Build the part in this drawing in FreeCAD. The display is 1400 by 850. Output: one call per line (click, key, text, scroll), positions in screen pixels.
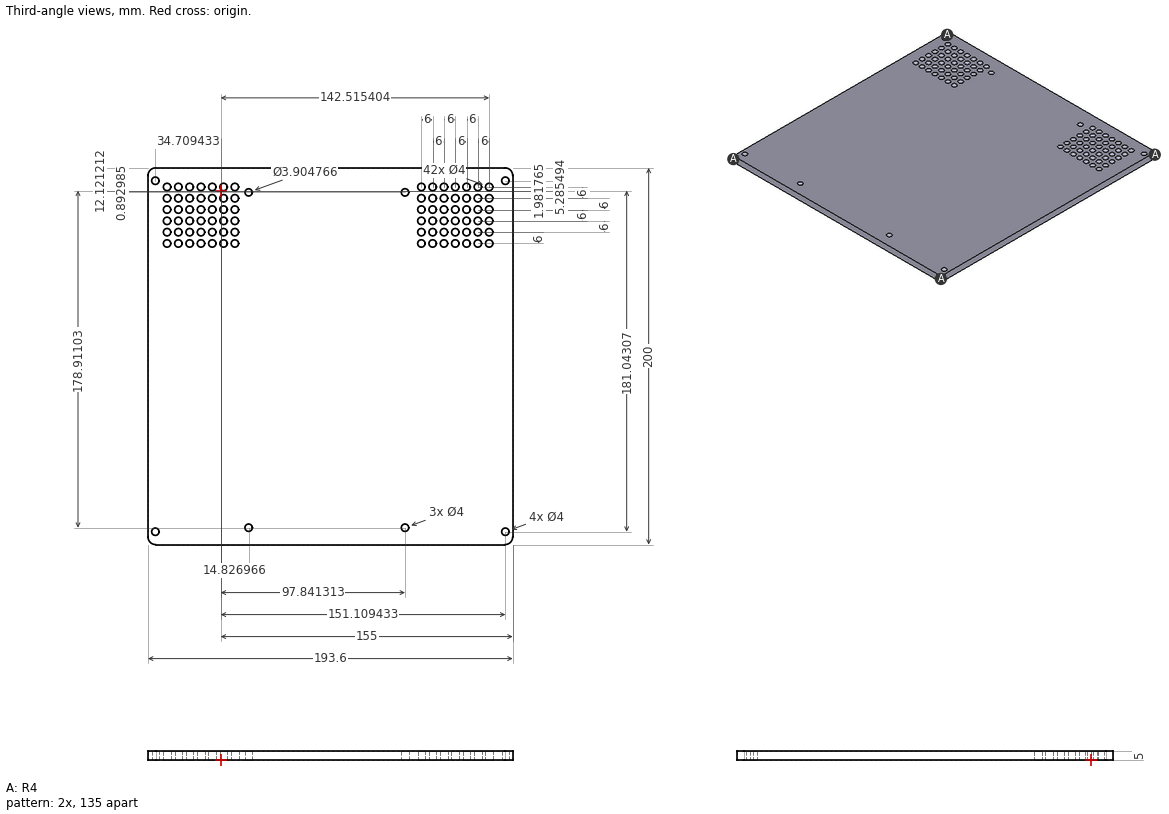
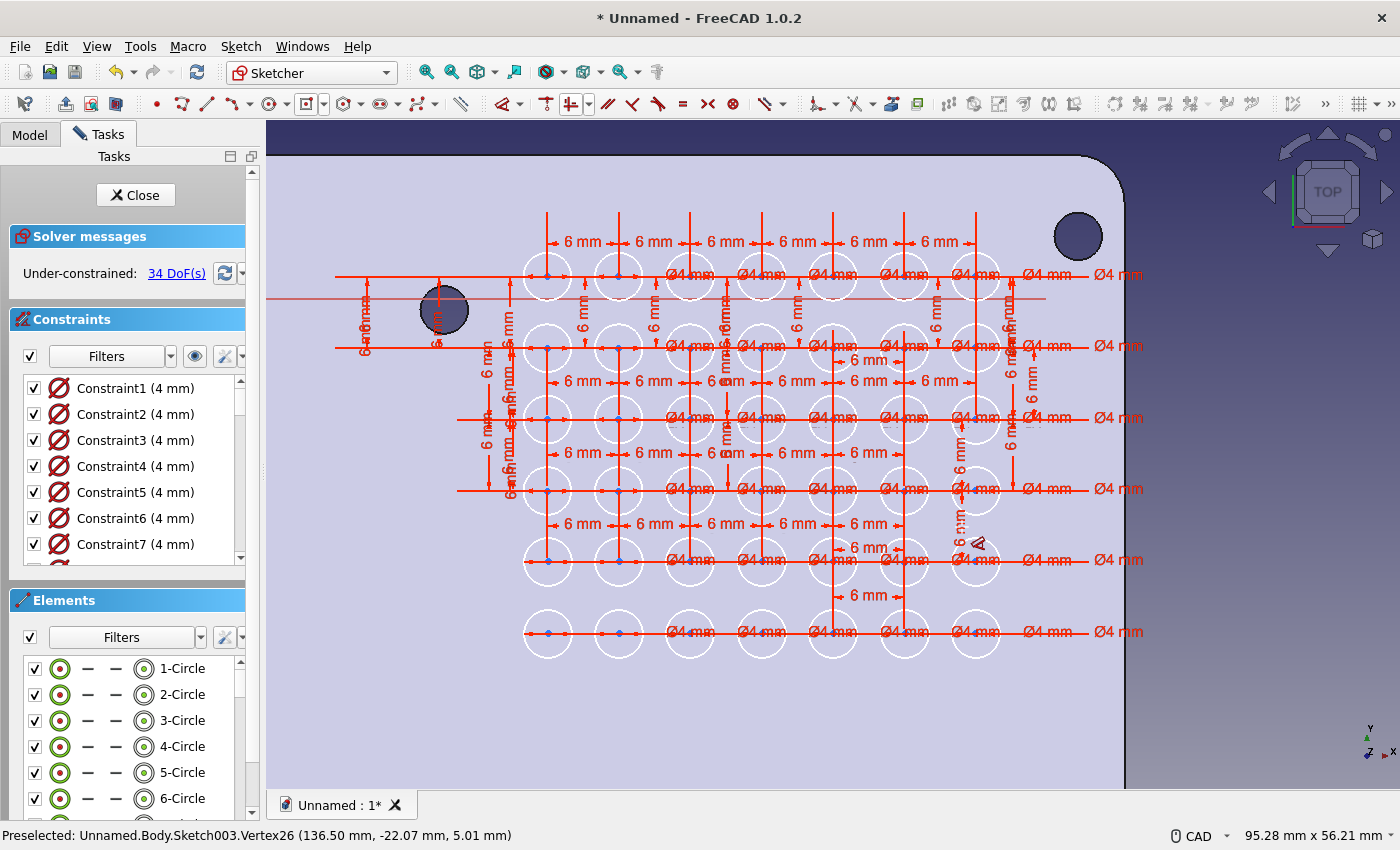
click(904, 562)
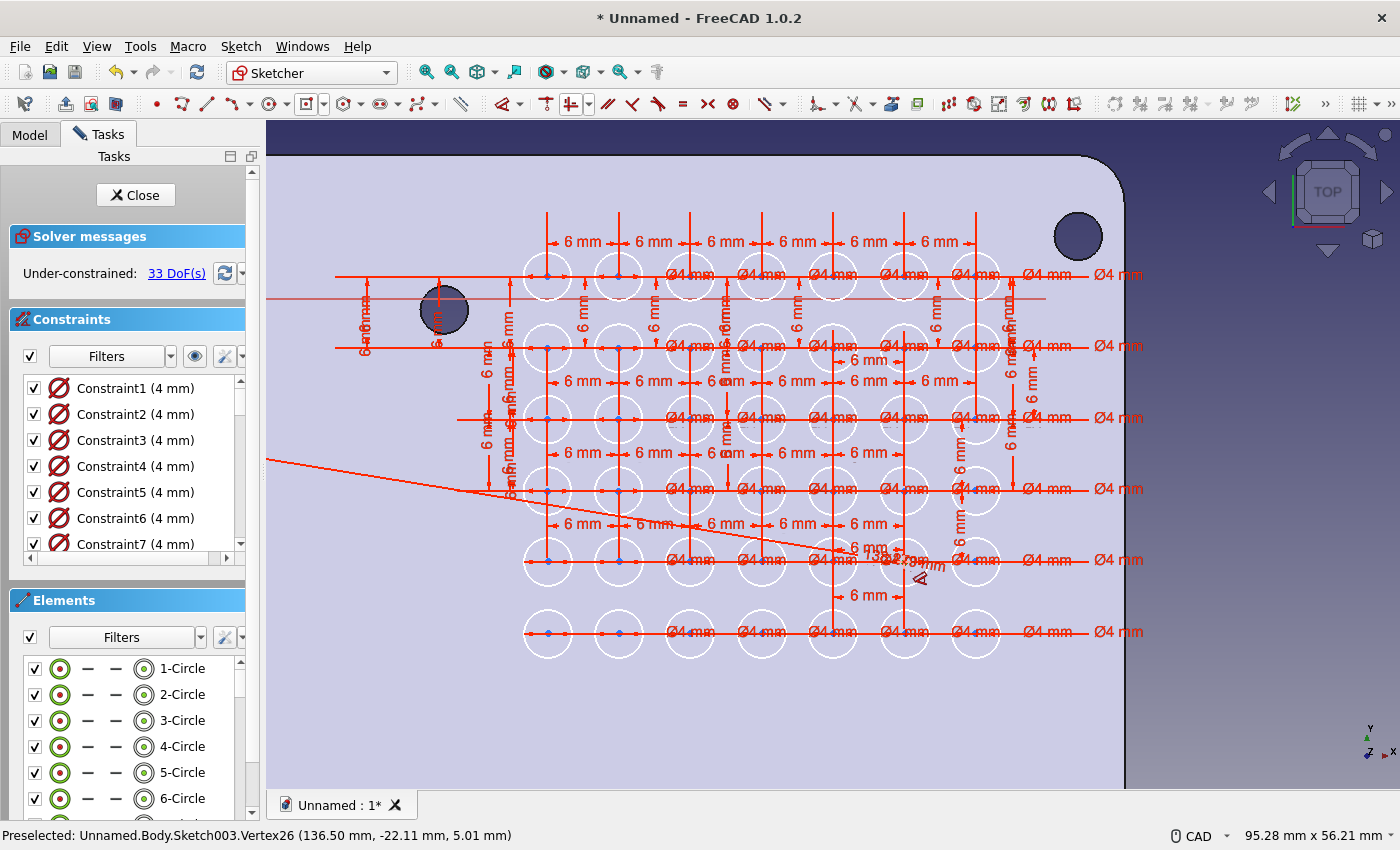
click(833, 562)
click(869, 620)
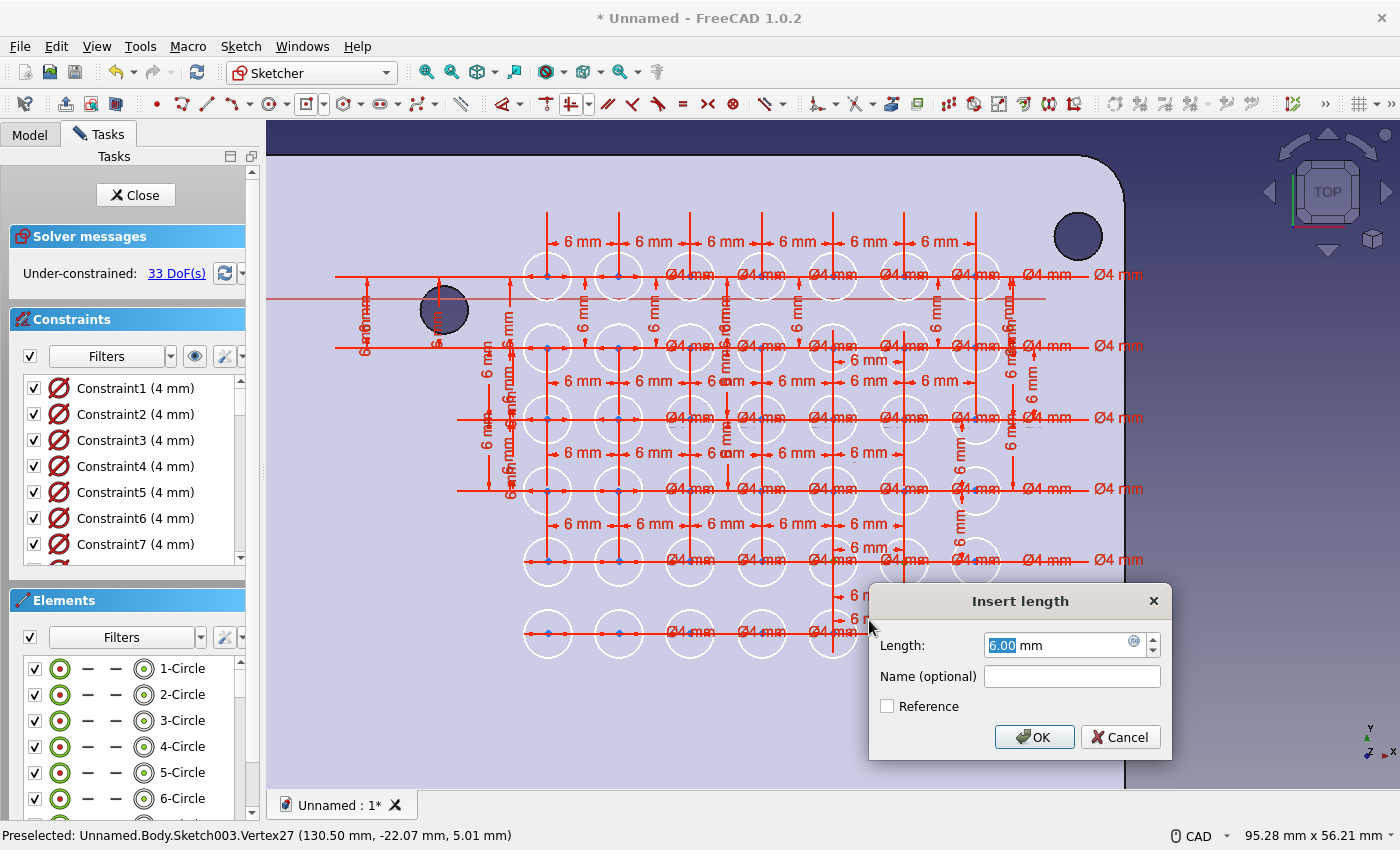
text(6)
key(Return)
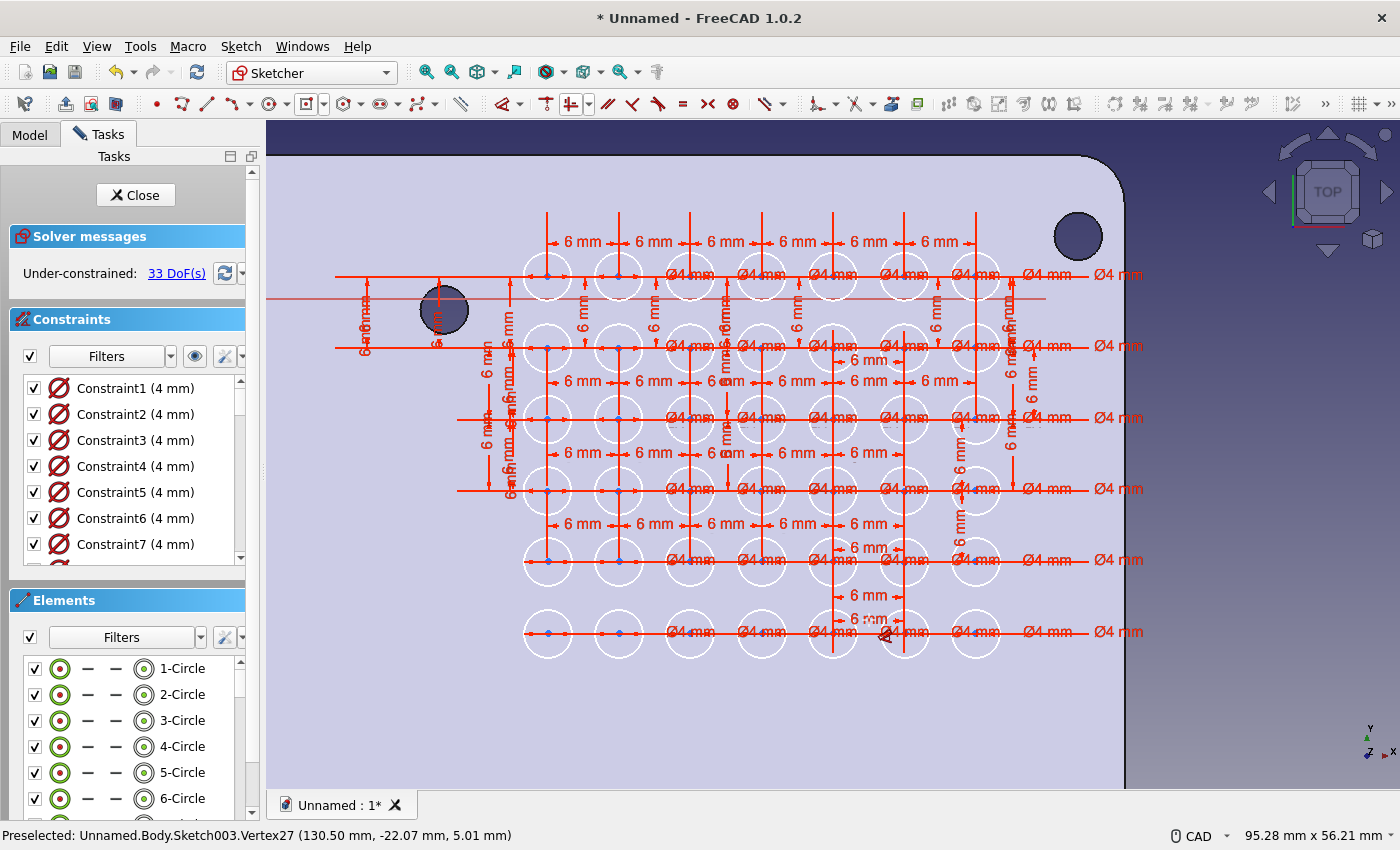
click(833, 491)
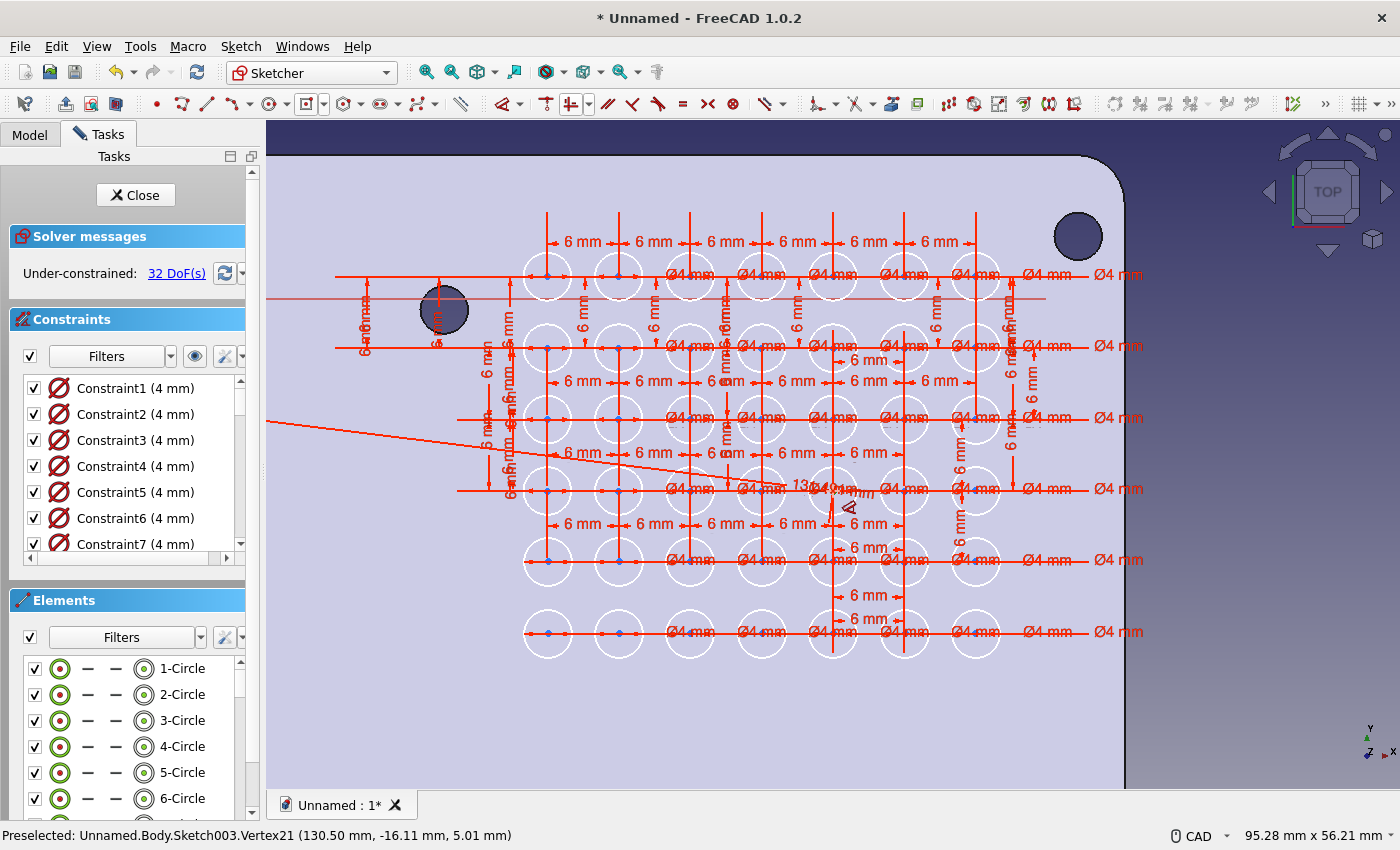
click(833, 562)
click(1013, 502)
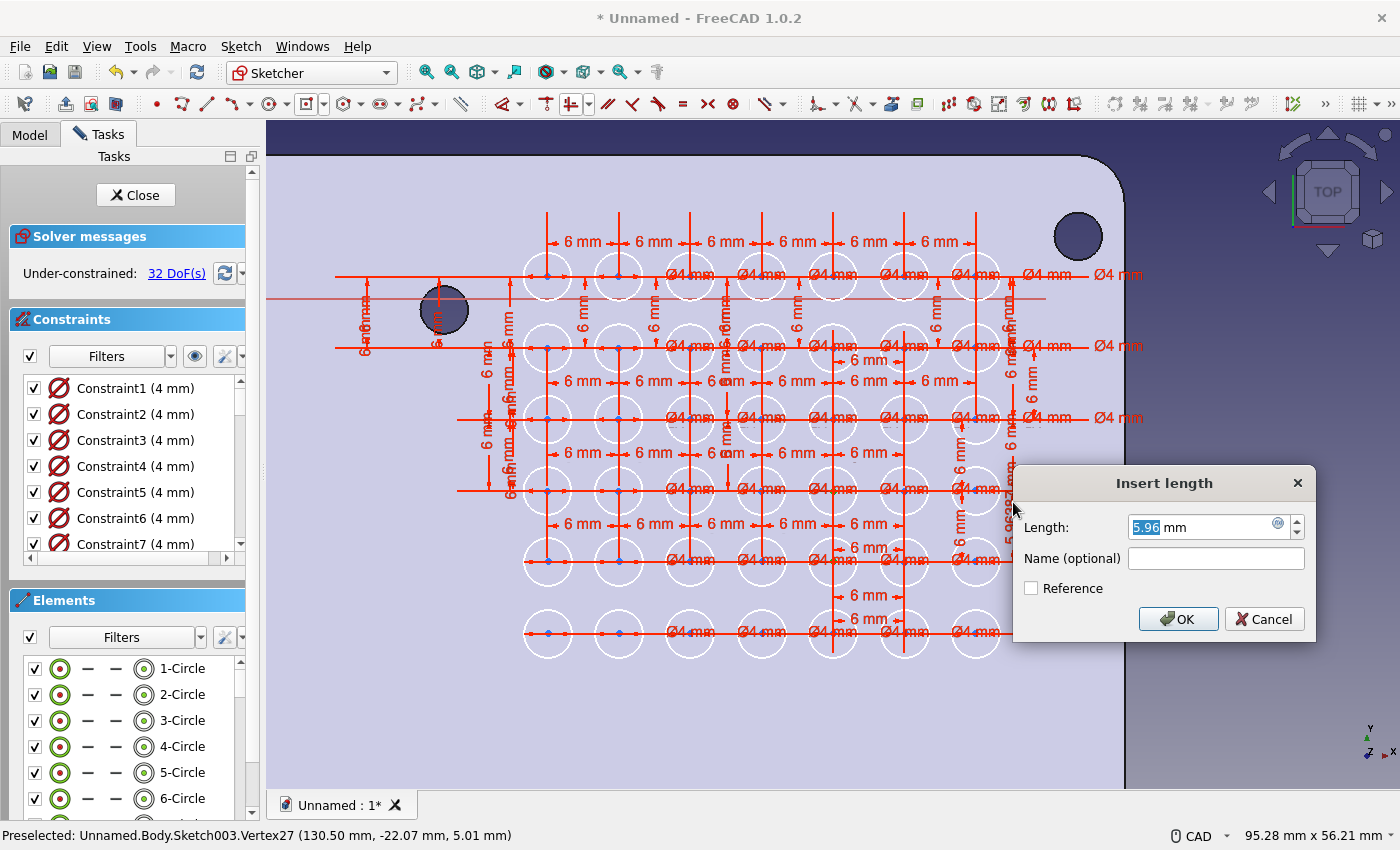
text(6)
key(Return)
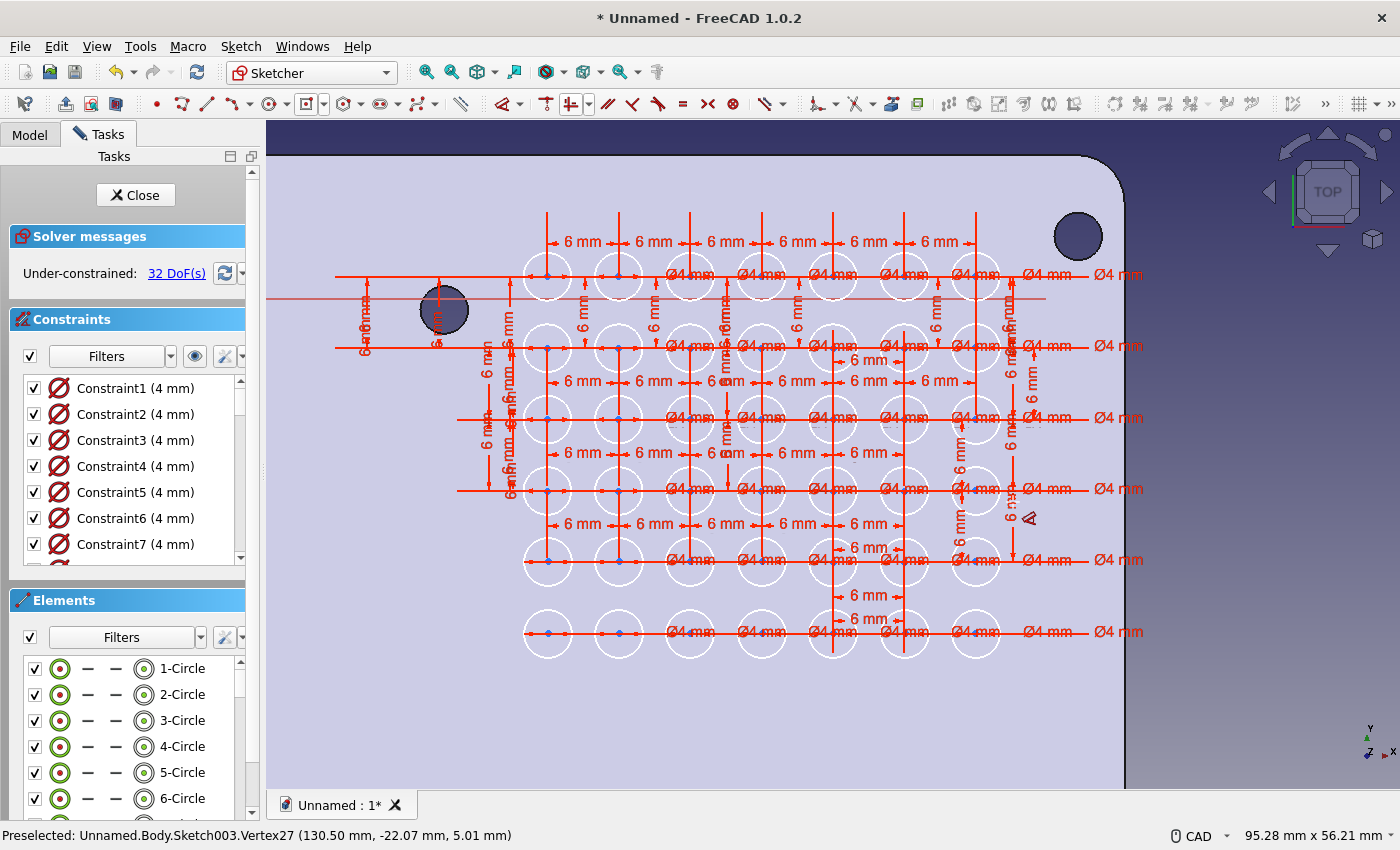
click(833, 562)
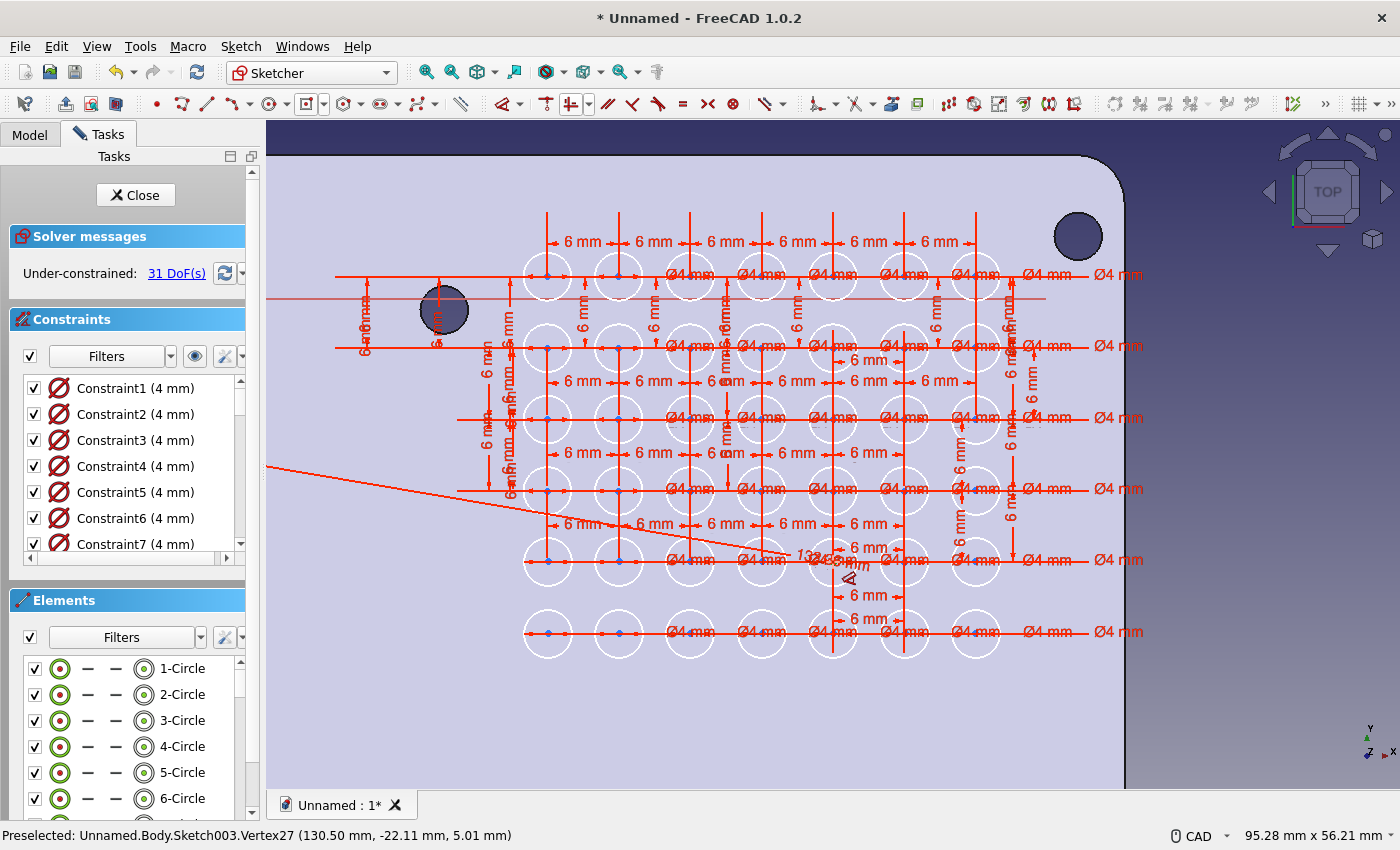
click(762, 562)
click(798, 596)